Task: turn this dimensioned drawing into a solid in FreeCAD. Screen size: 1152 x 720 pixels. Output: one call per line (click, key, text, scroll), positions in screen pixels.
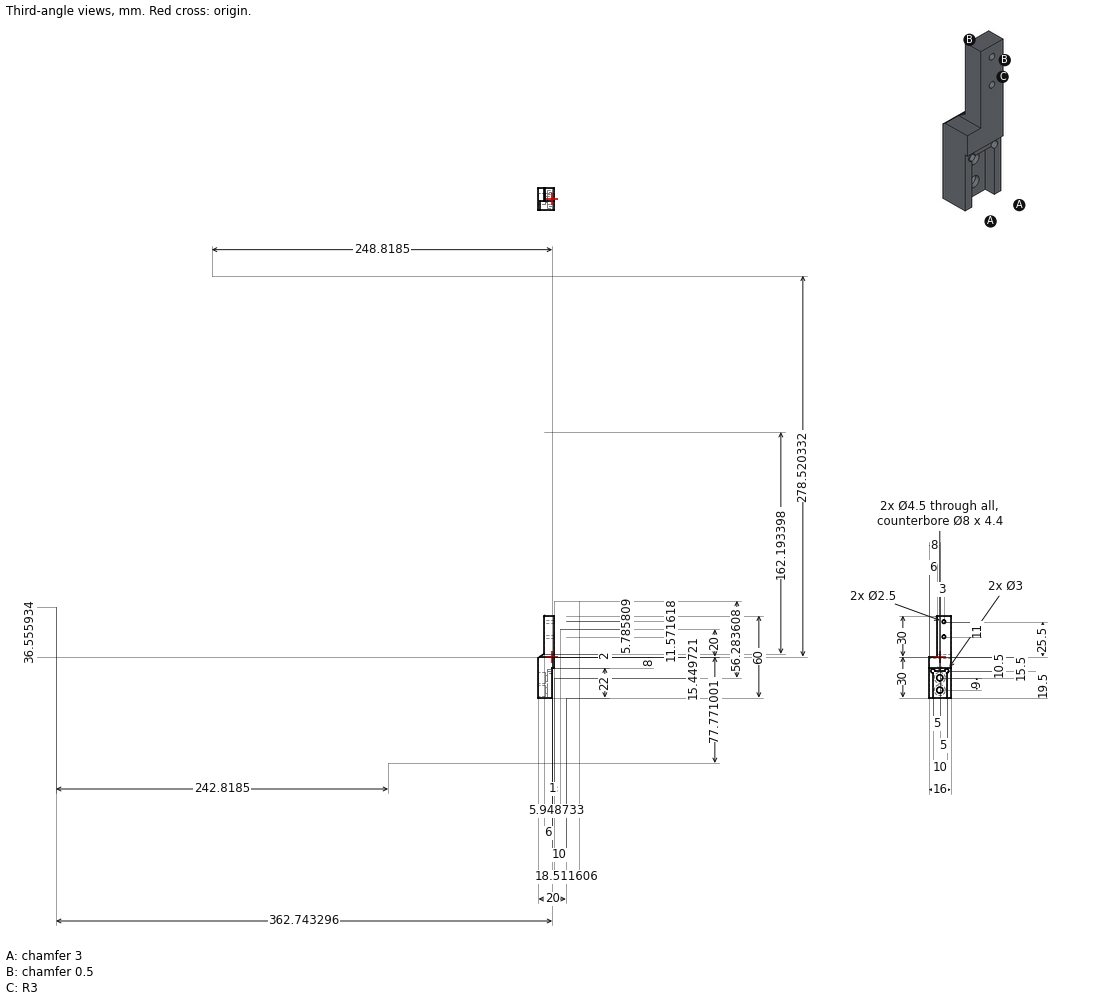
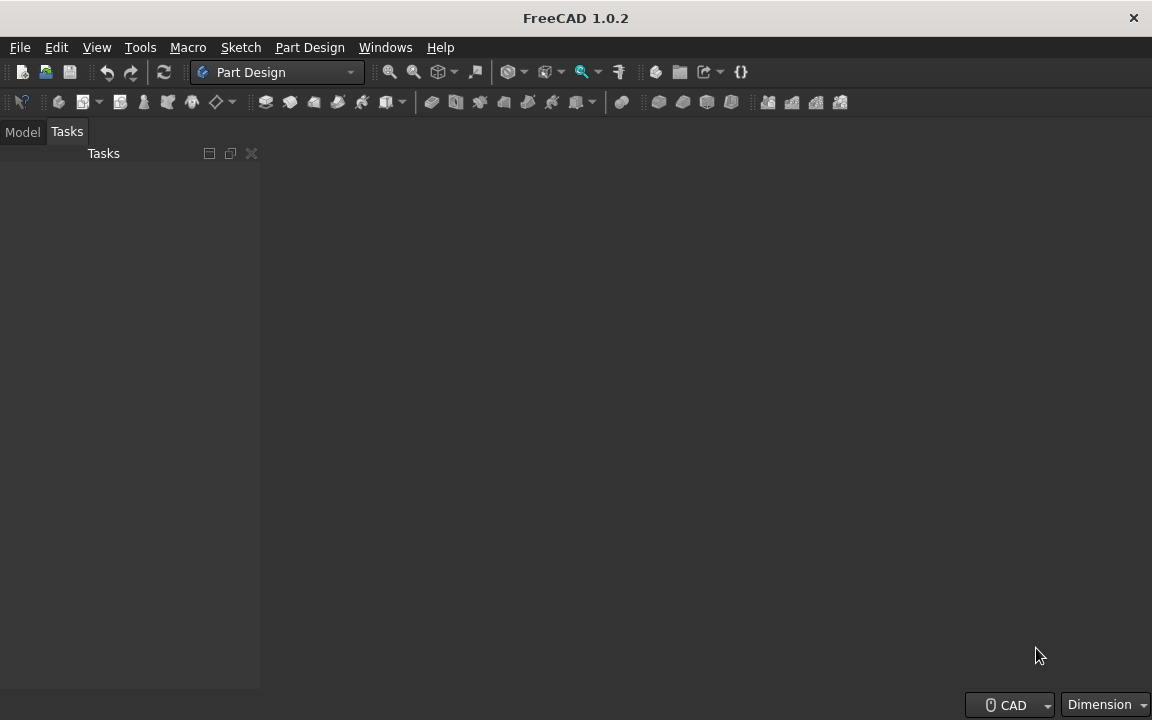
click(22, 72)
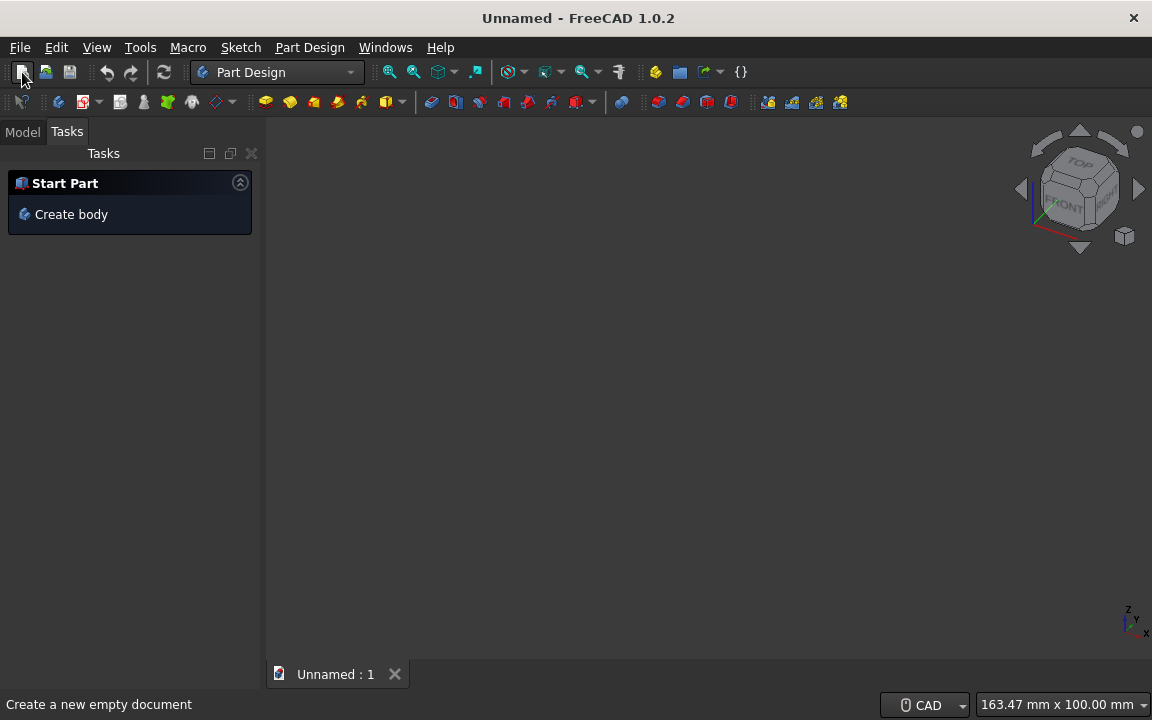
click(84, 102)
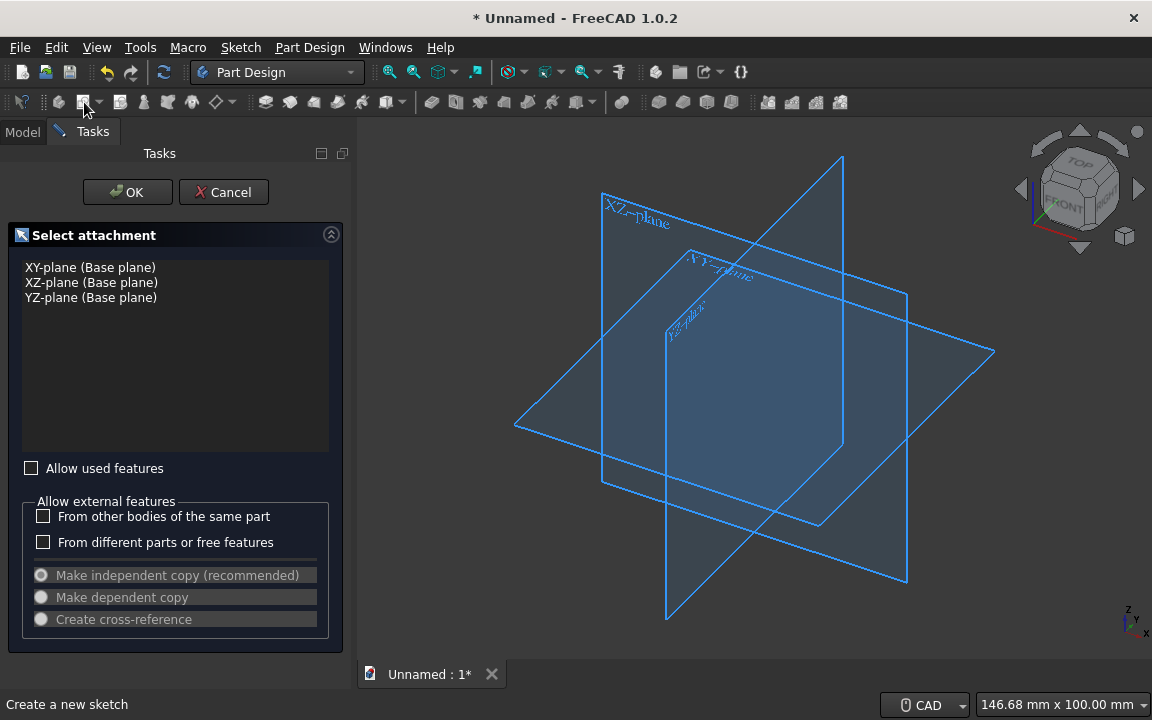
click(82, 282)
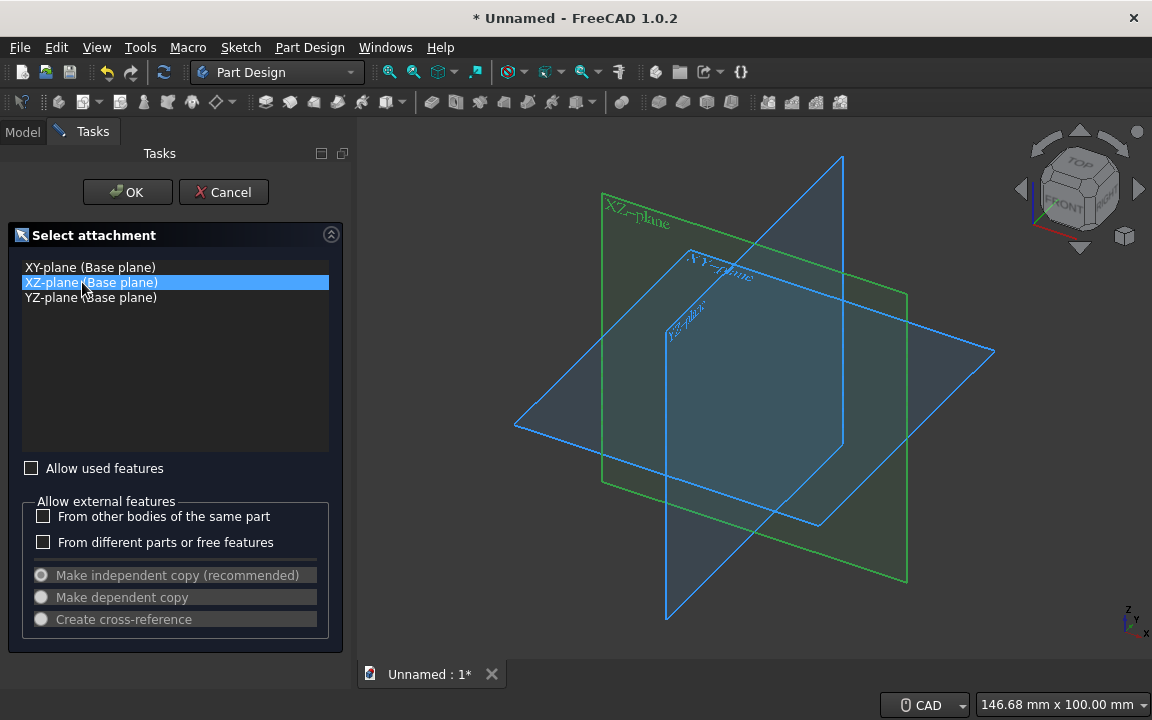
click(128, 192)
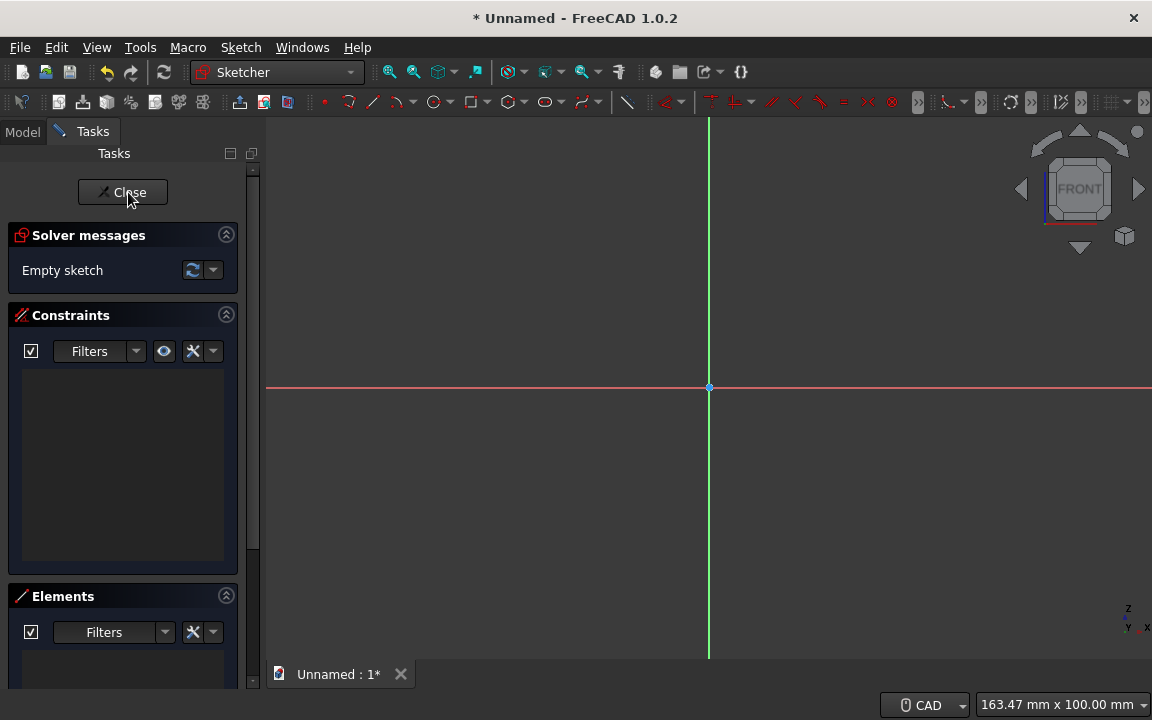
key(g)
key(v)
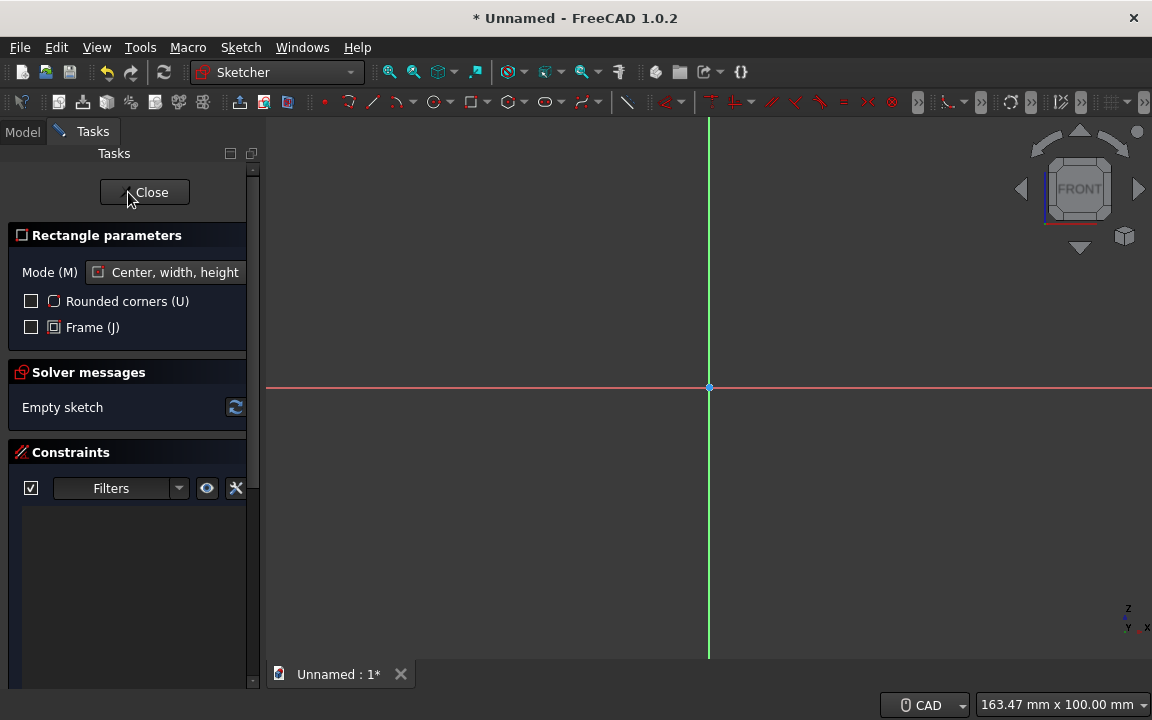
click(709, 388)
click(763, 225)
key(Escape)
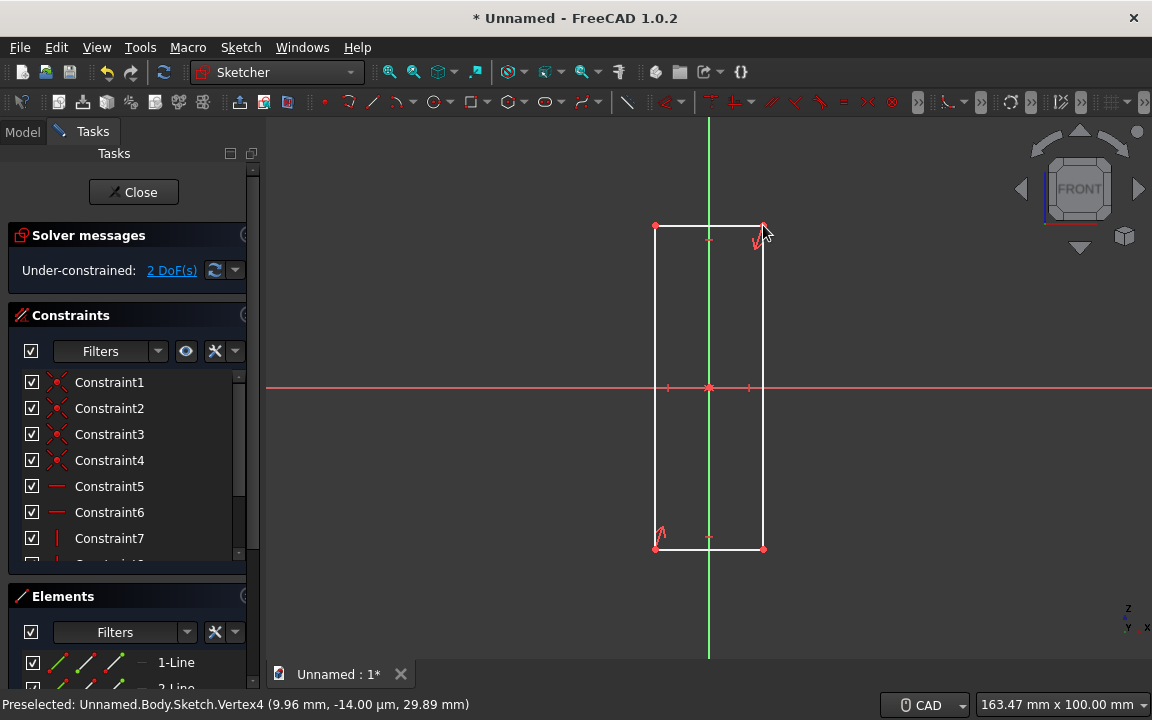
click(666, 102)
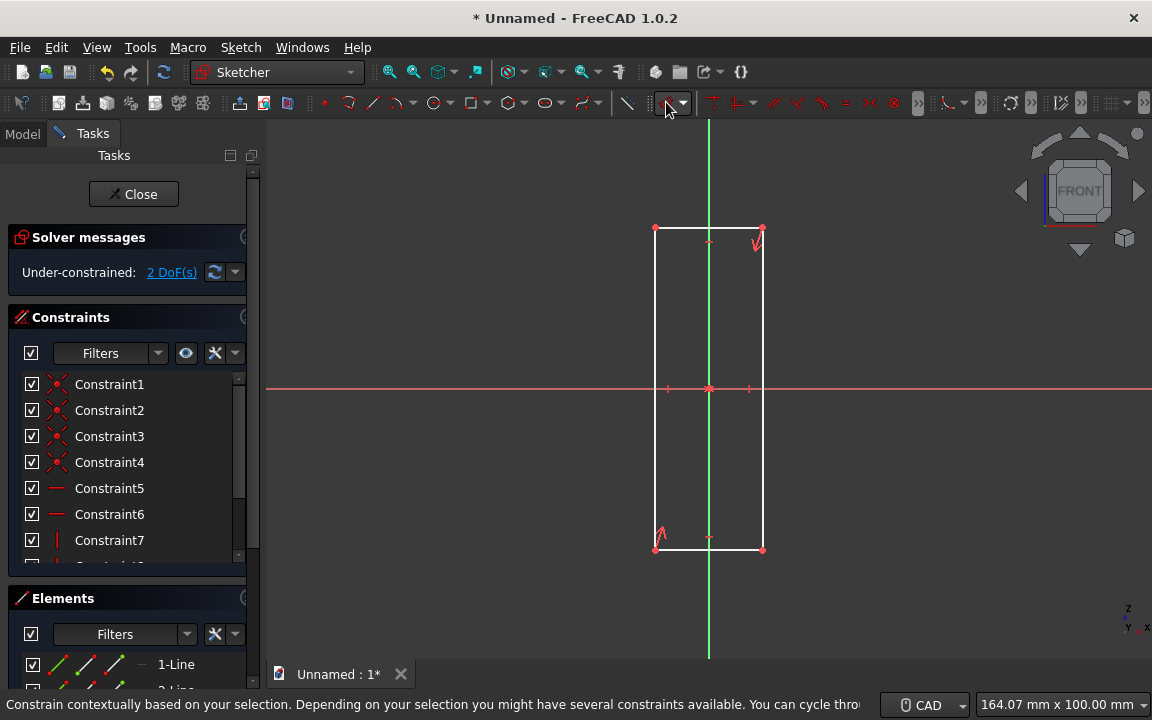
click(687, 550)
click(684, 584)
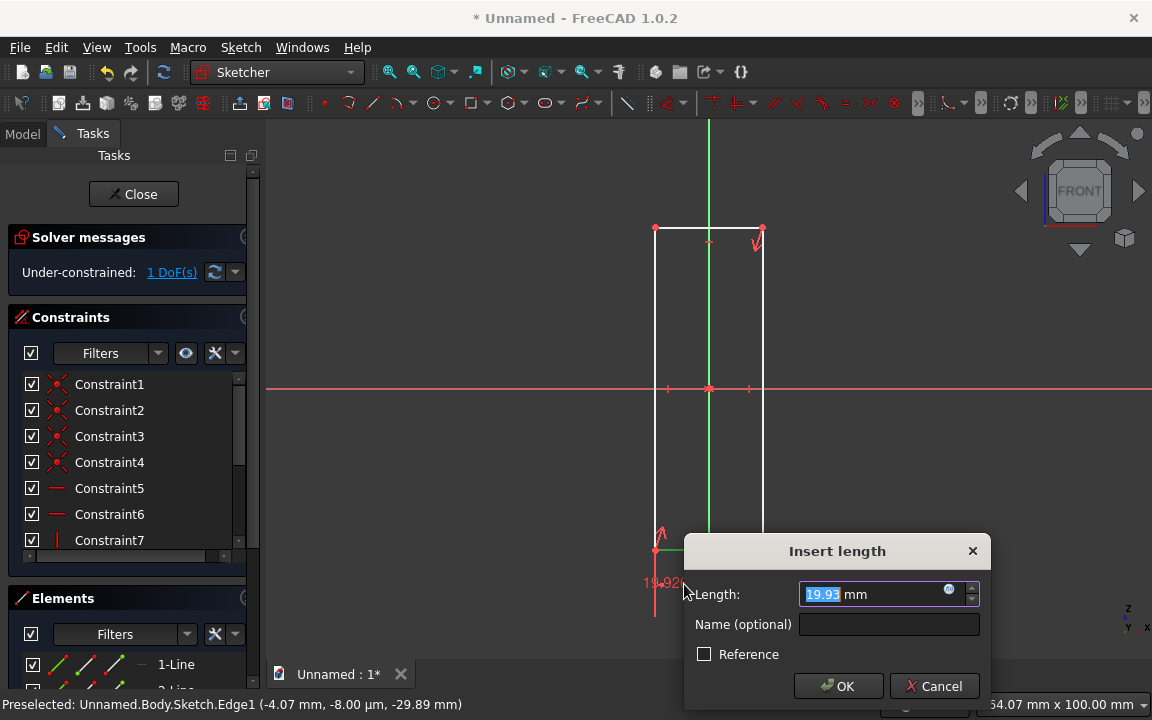
text(20)
key(Return)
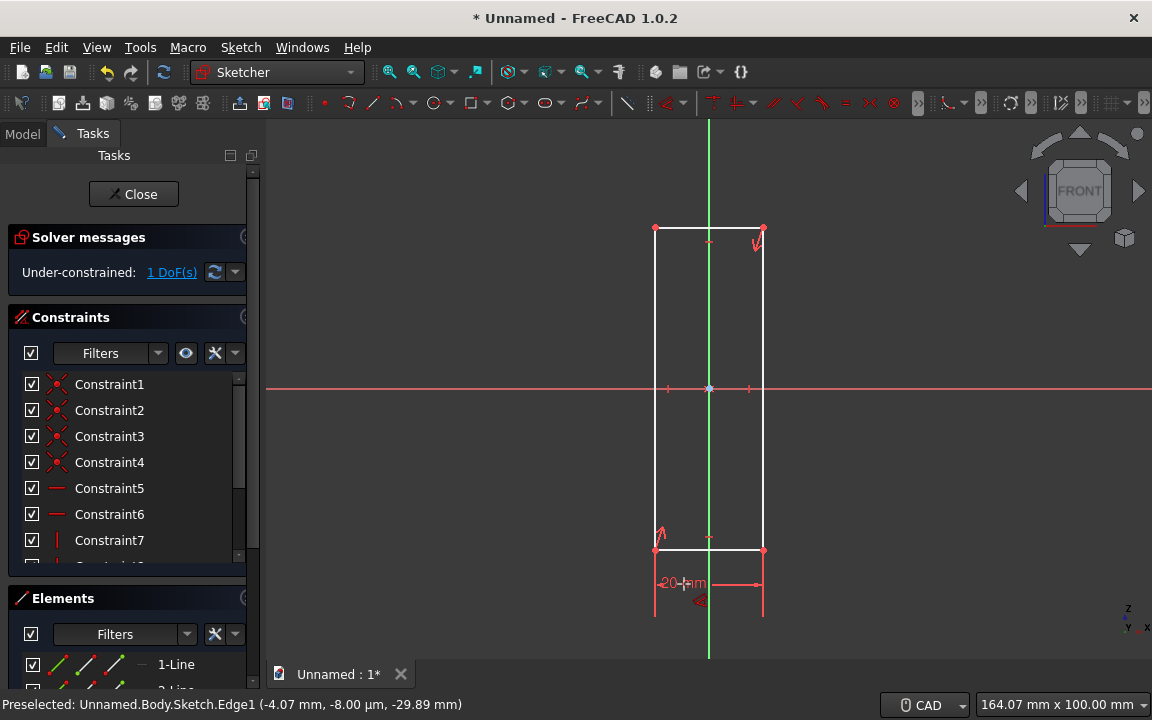
click(763, 454)
click(797, 315)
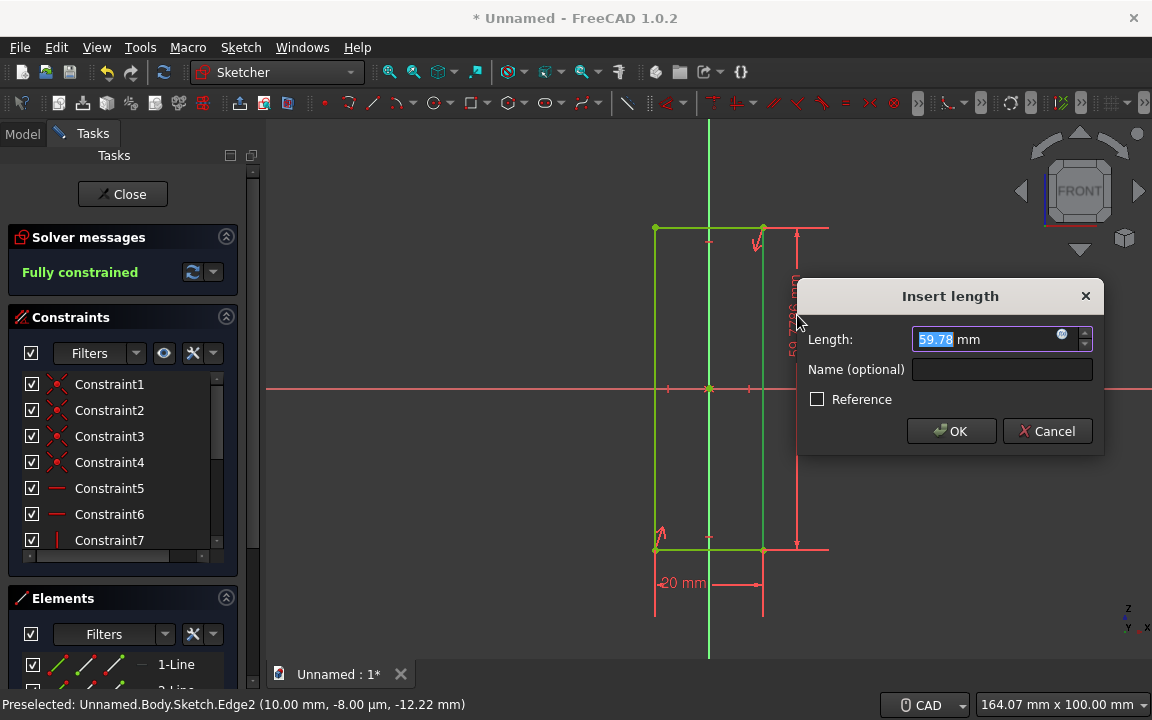
text(60)
key(Return)
key(Escape)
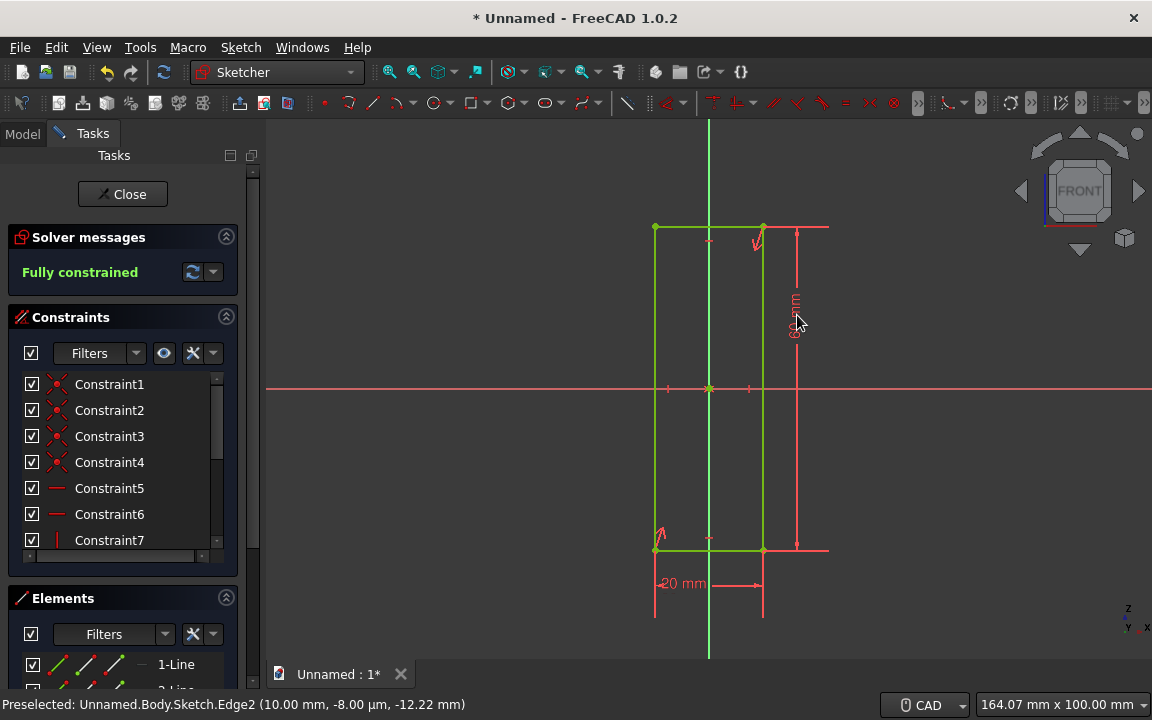
click(123, 194)